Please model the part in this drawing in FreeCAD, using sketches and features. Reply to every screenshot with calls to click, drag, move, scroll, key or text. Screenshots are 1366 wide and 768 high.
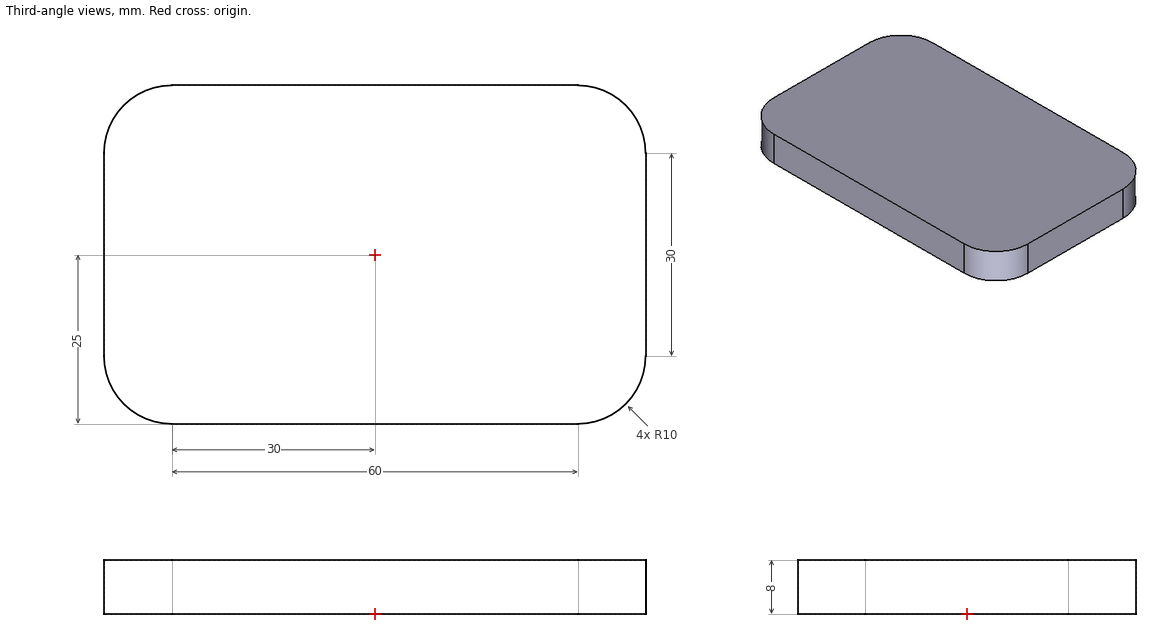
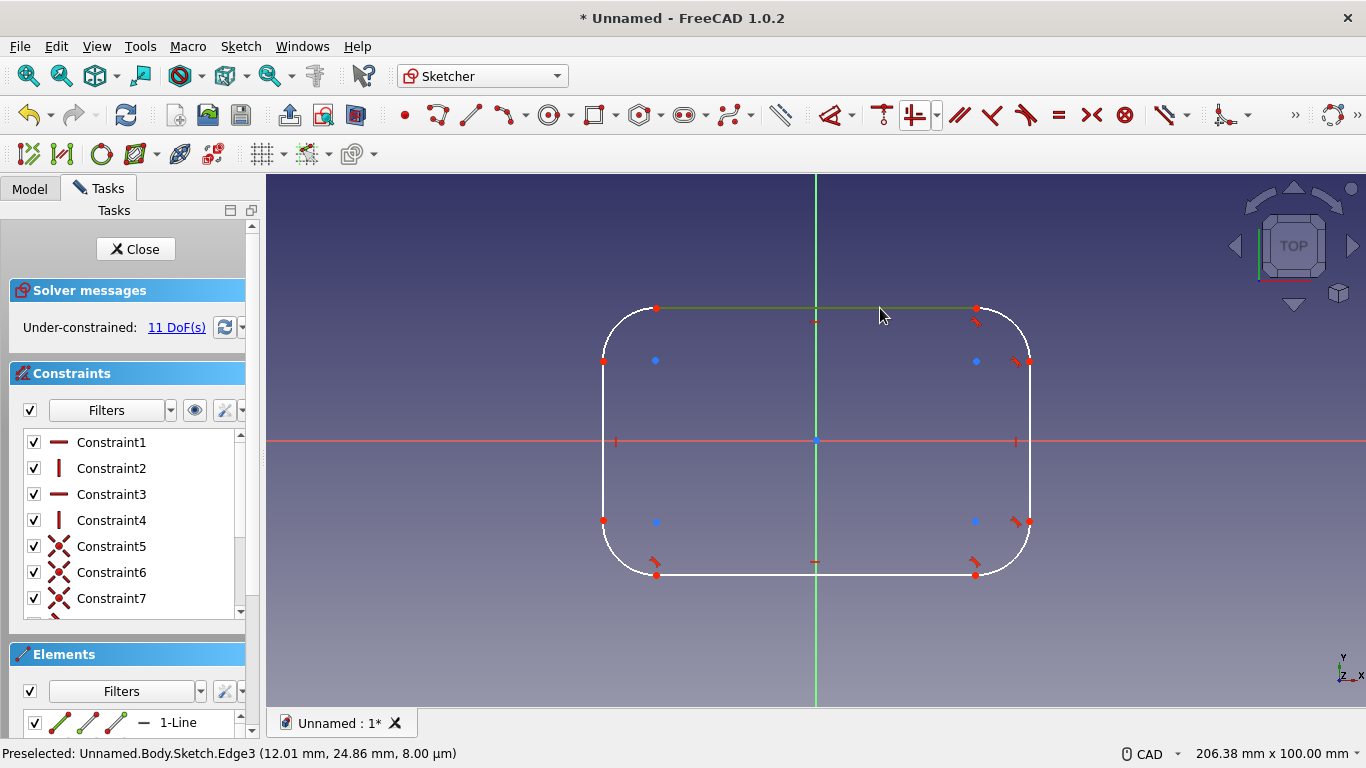
click(632, 314)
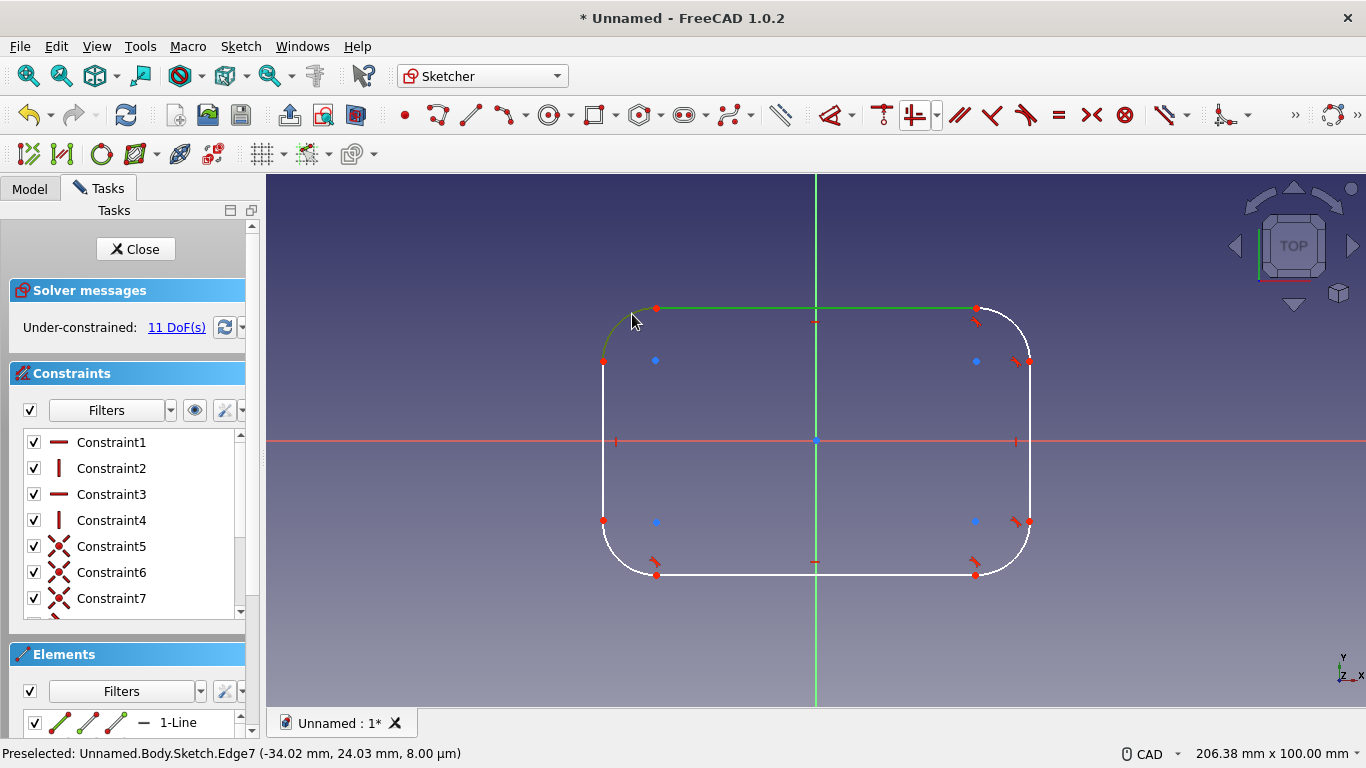
click(1026, 116)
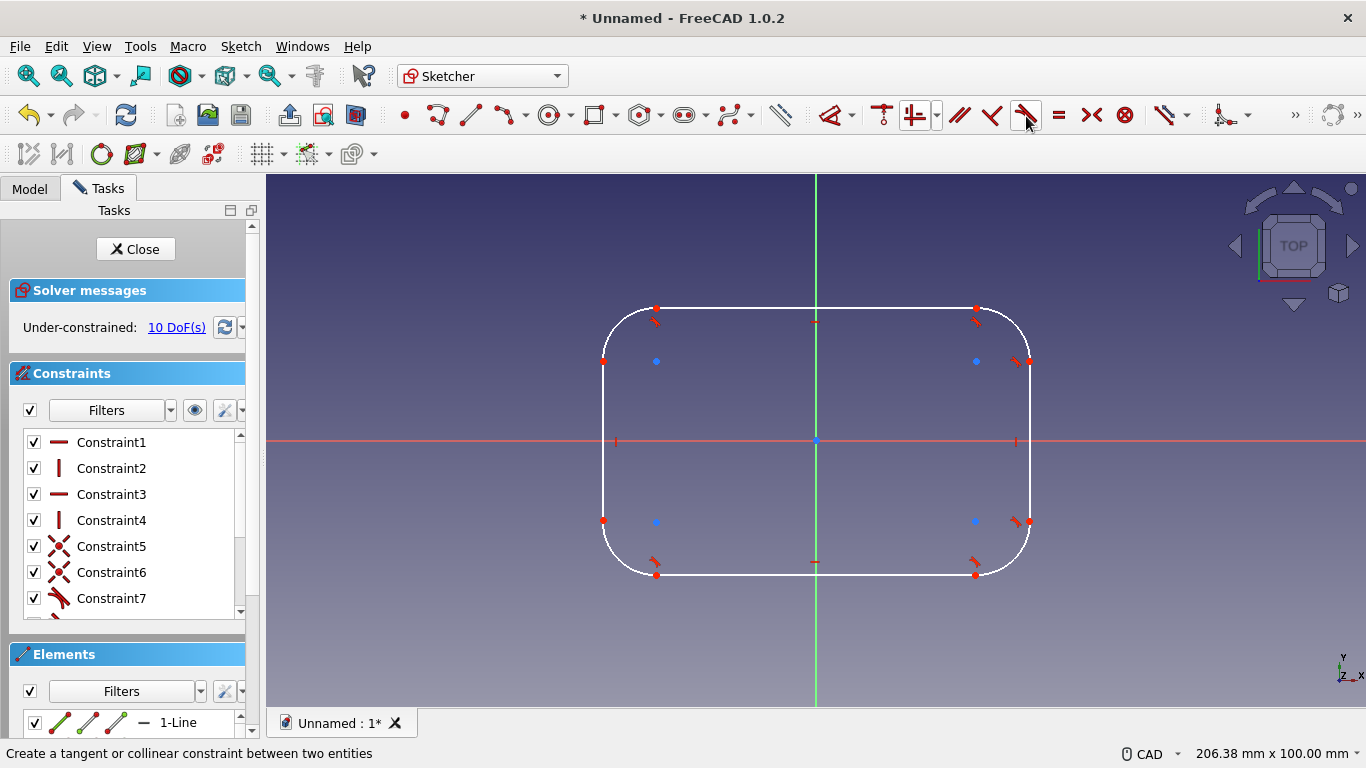
click(603, 410)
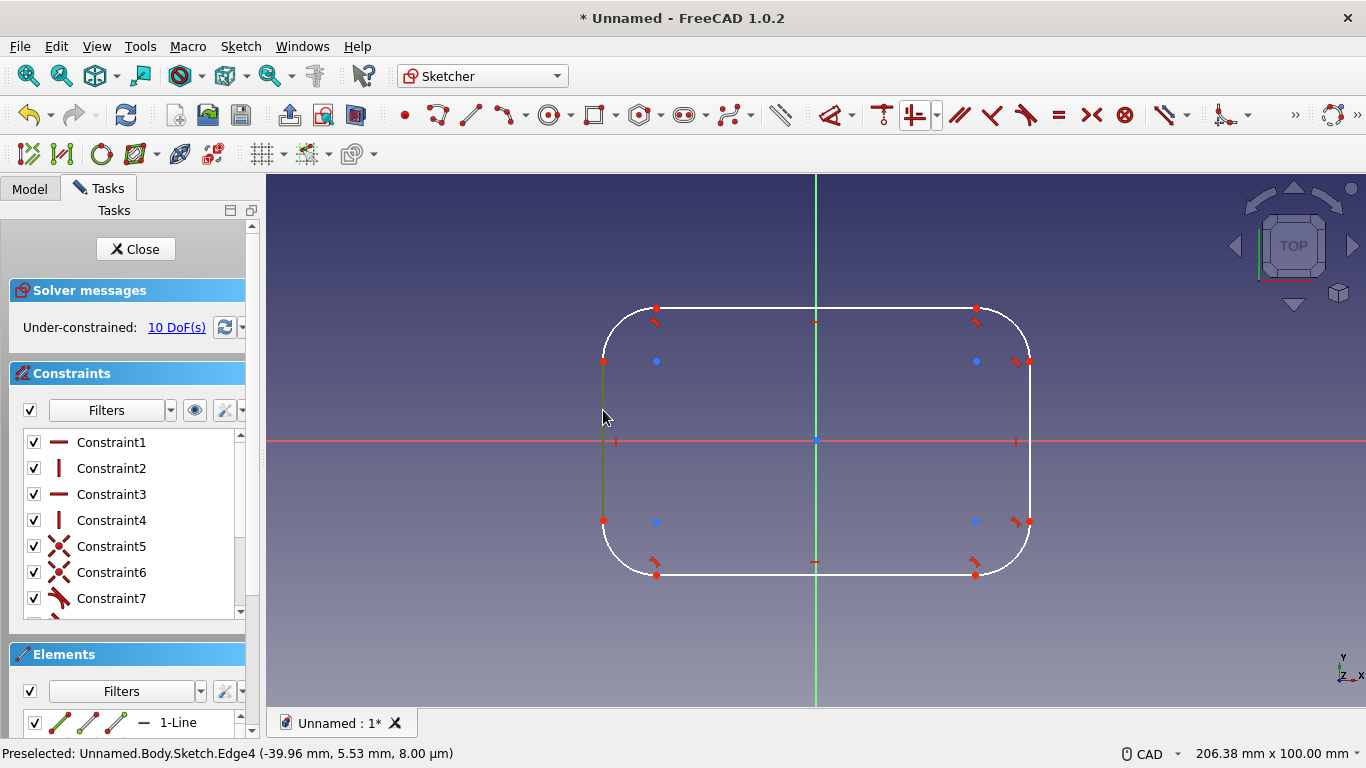
click(632, 314)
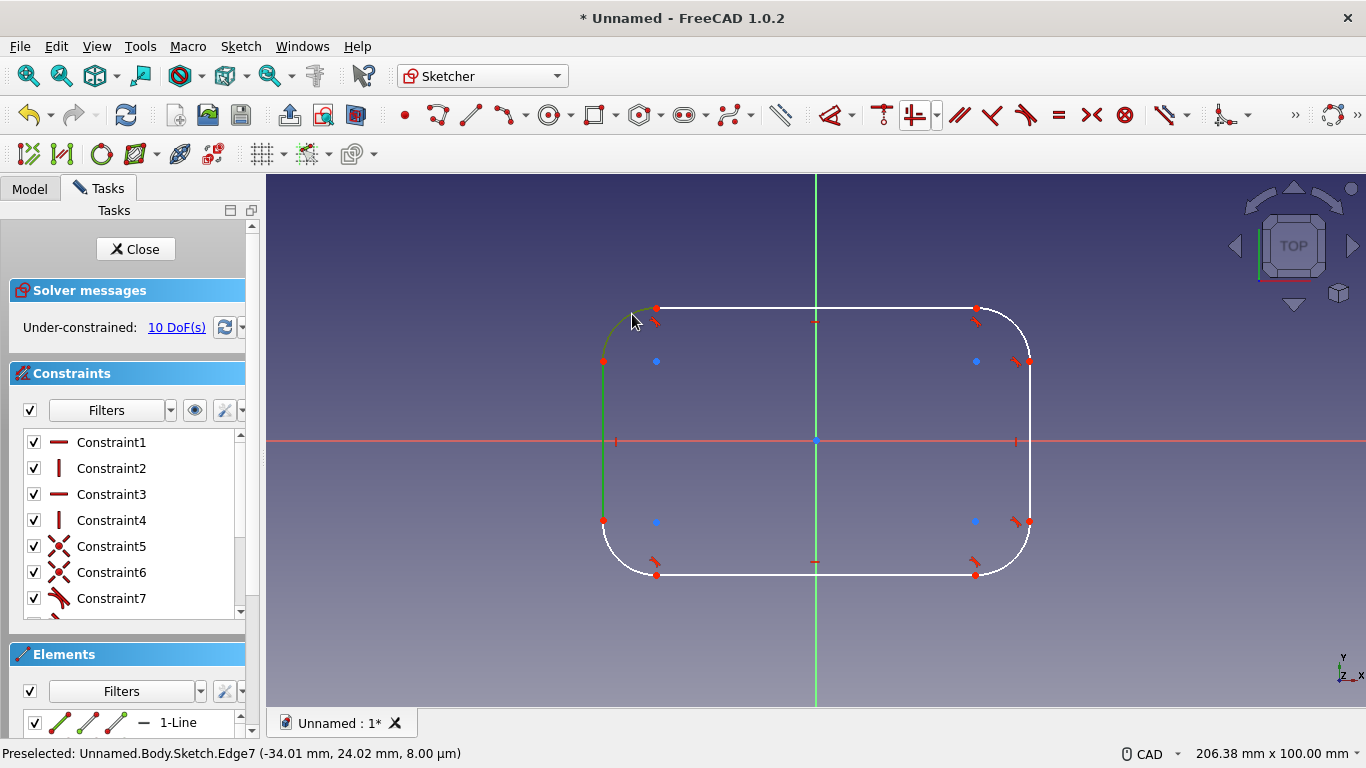
key(t)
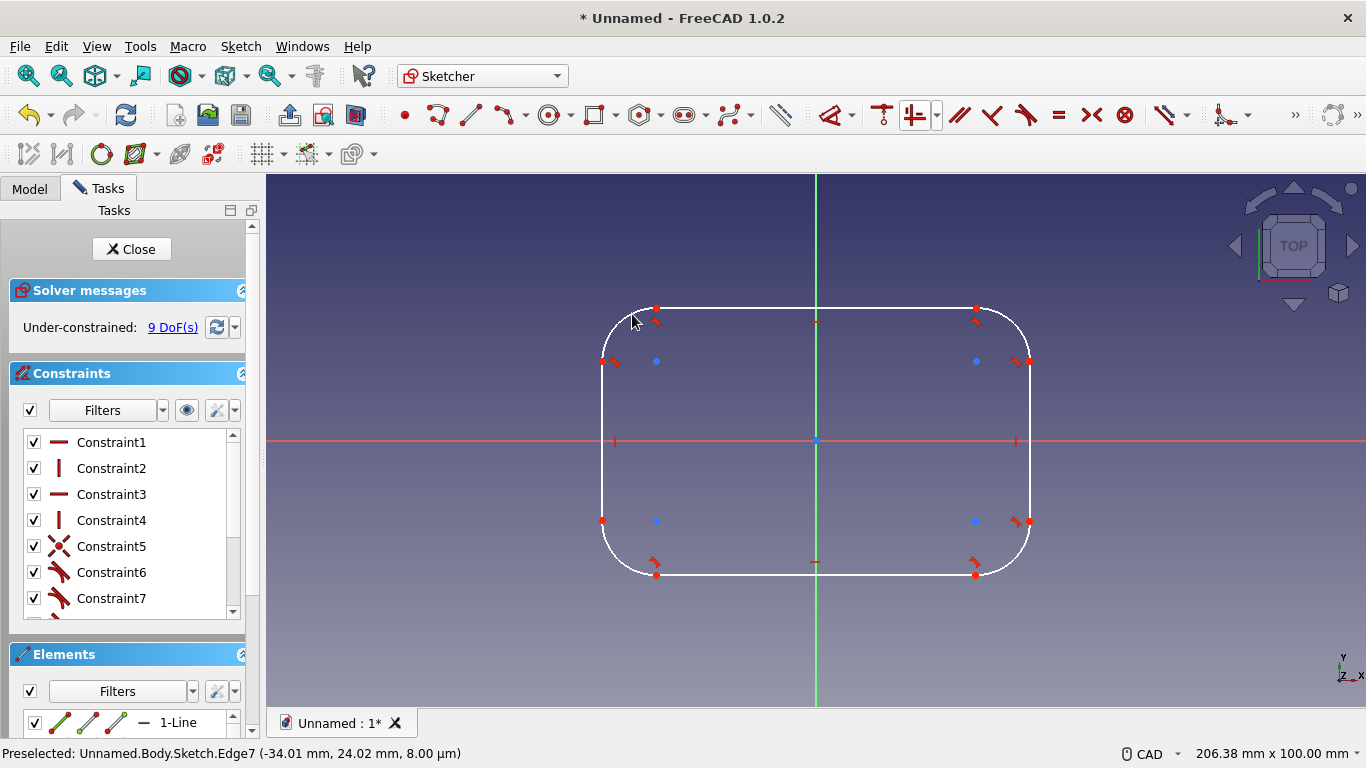
click(602, 410)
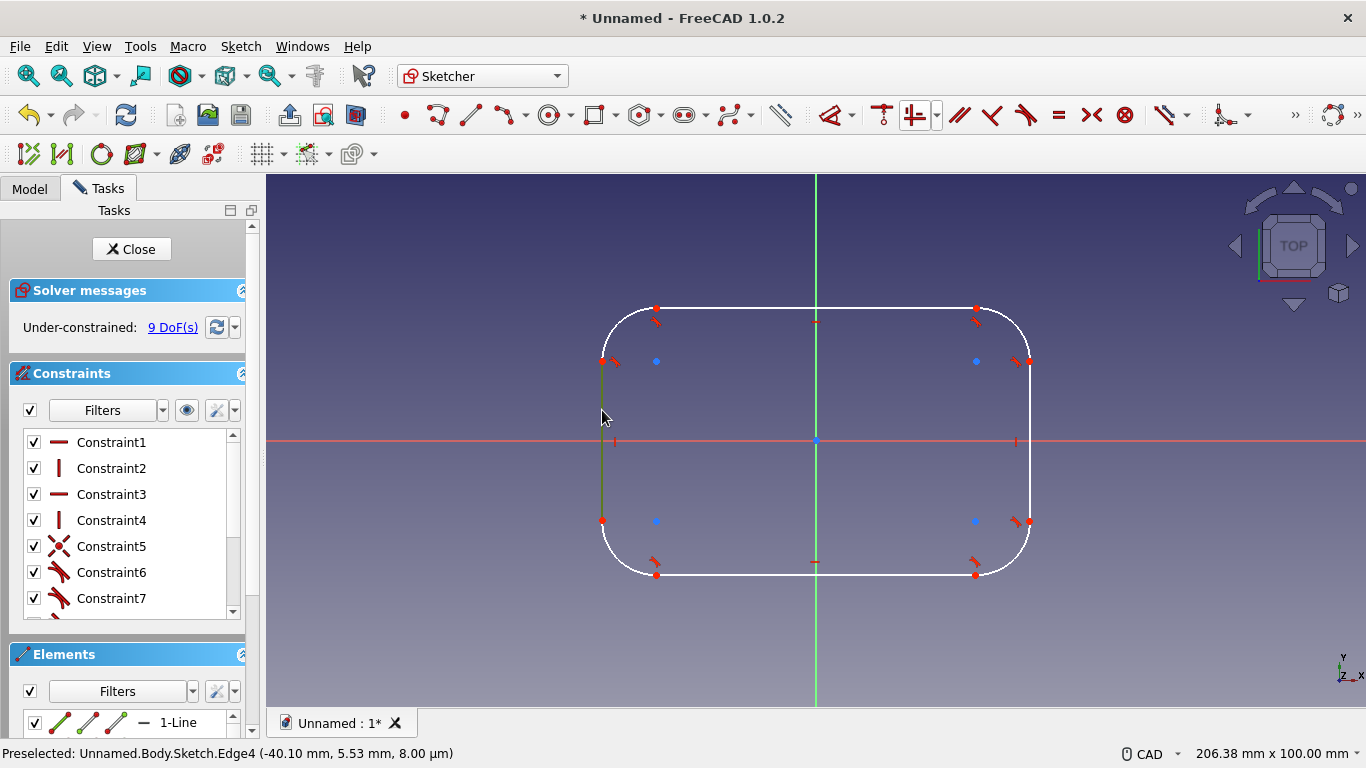
click(608, 546)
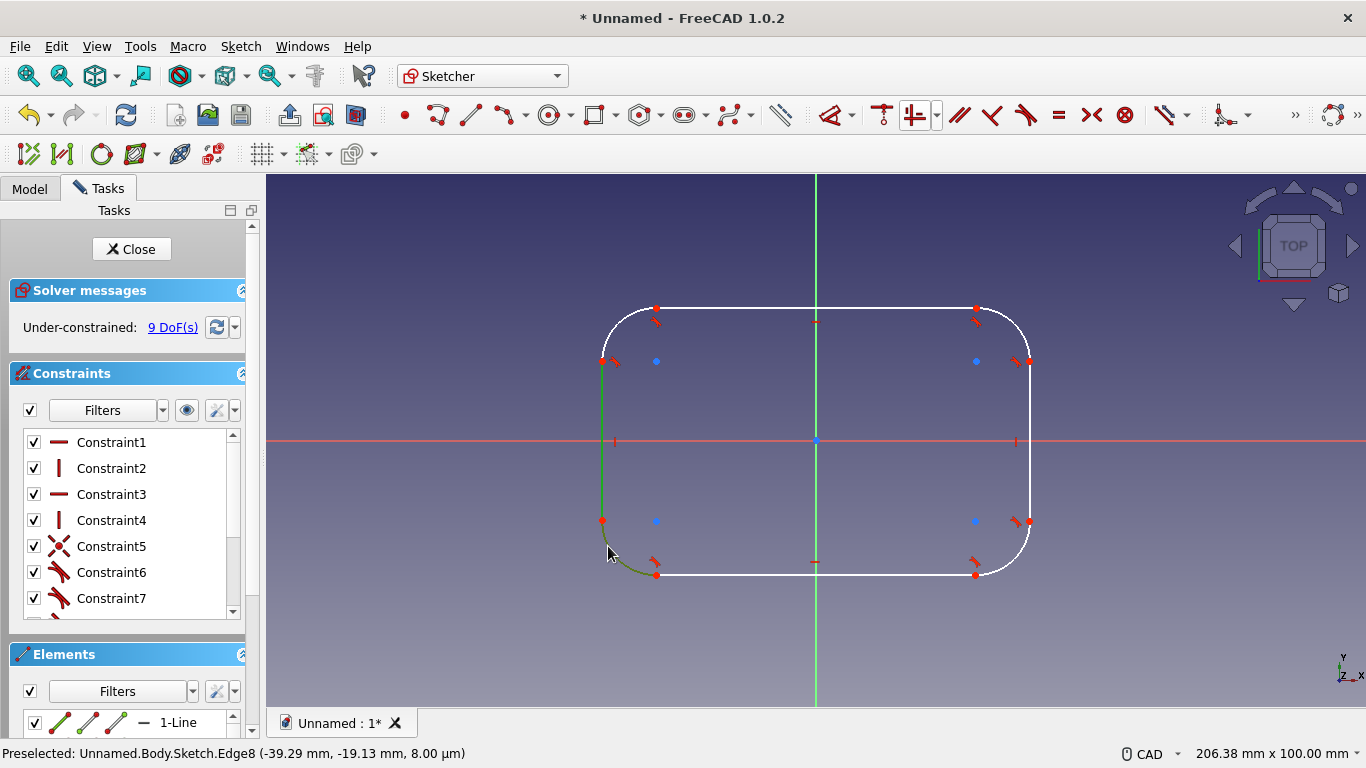
key(t)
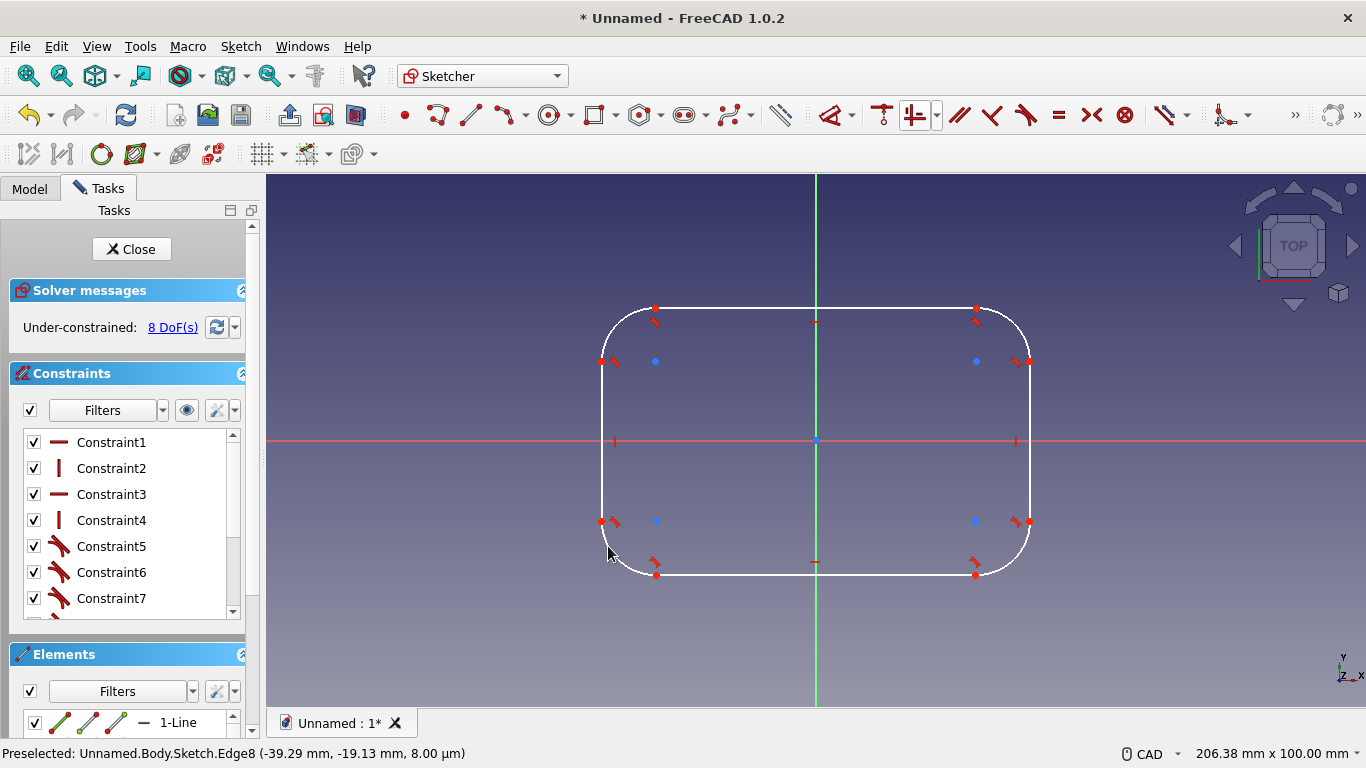
click(1000, 569)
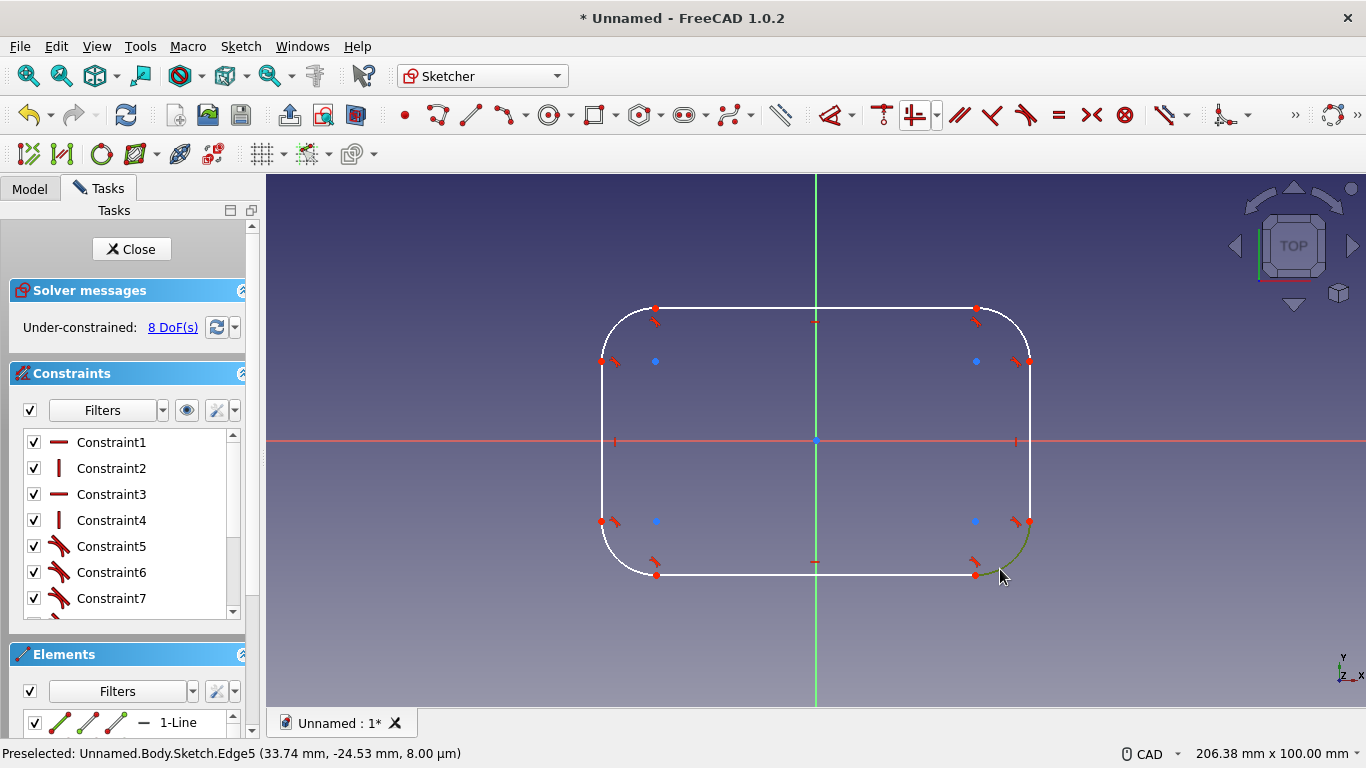
click(1024, 337)